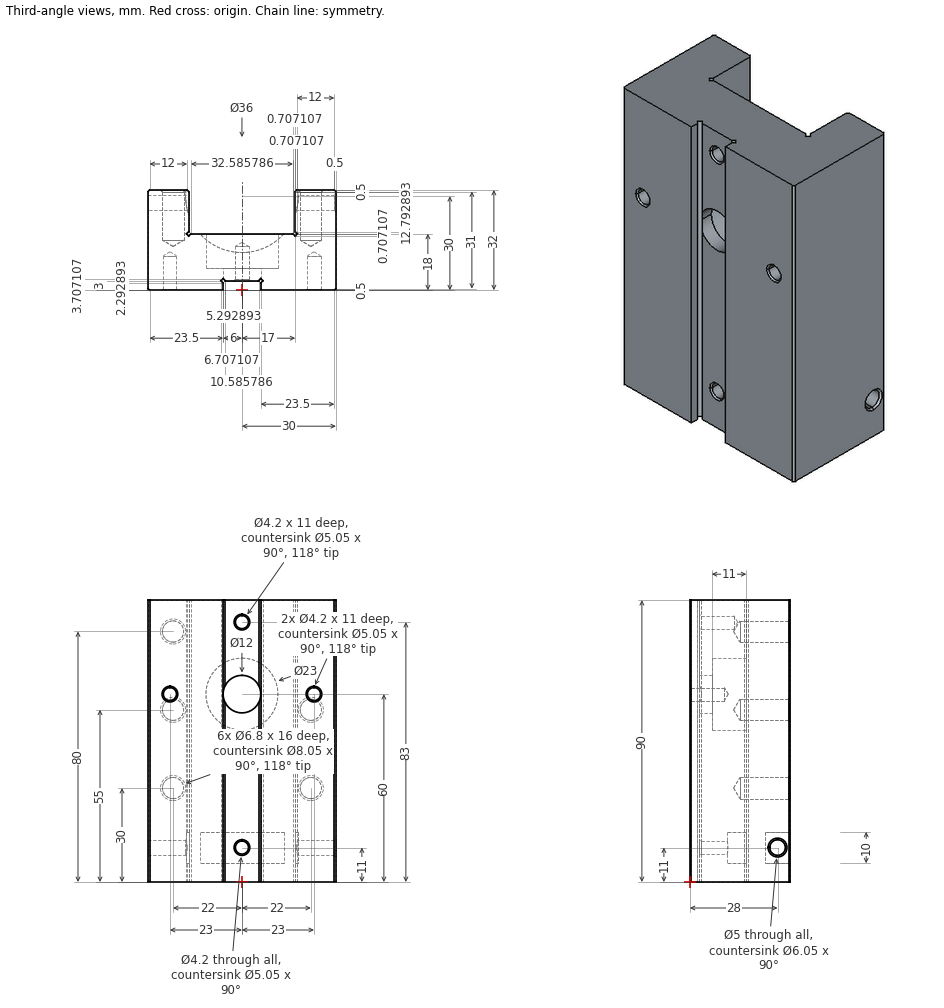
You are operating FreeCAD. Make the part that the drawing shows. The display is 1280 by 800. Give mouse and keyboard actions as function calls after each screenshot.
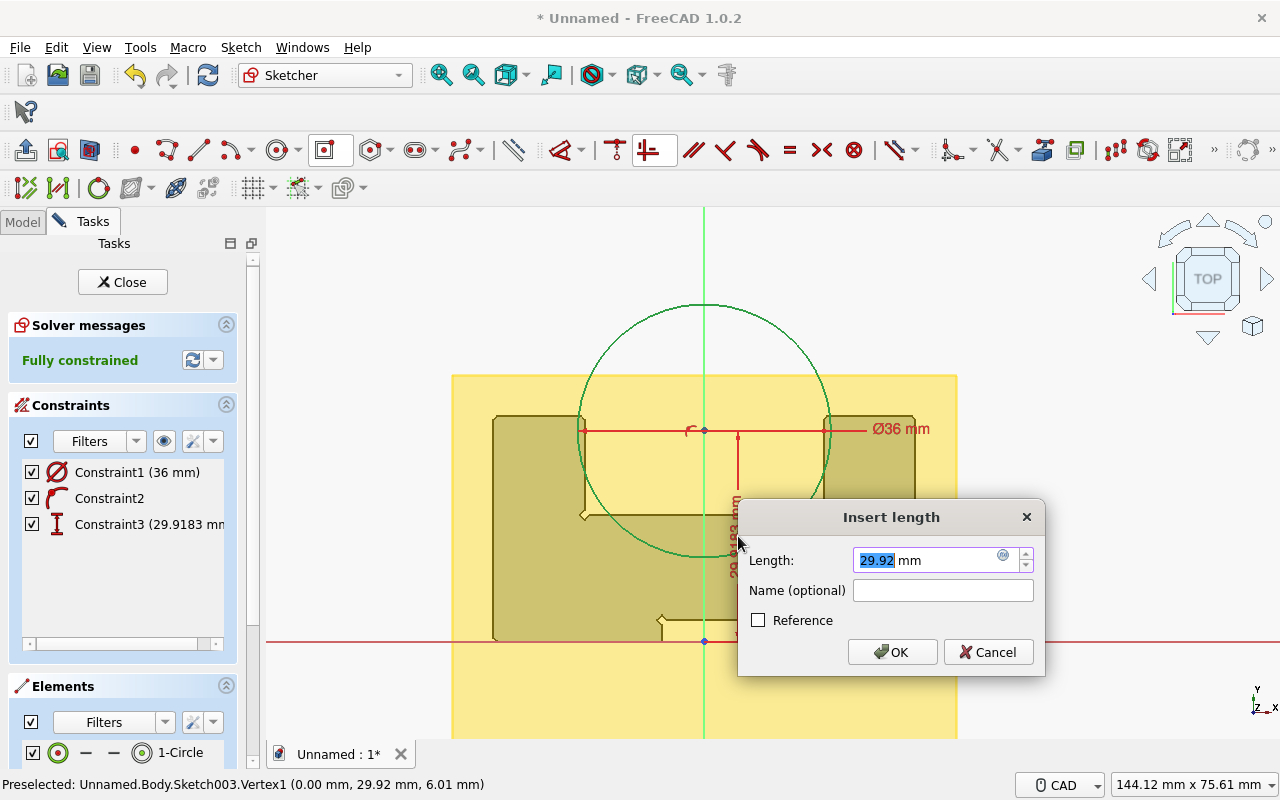
text(30)
key(Return)
key(Escape)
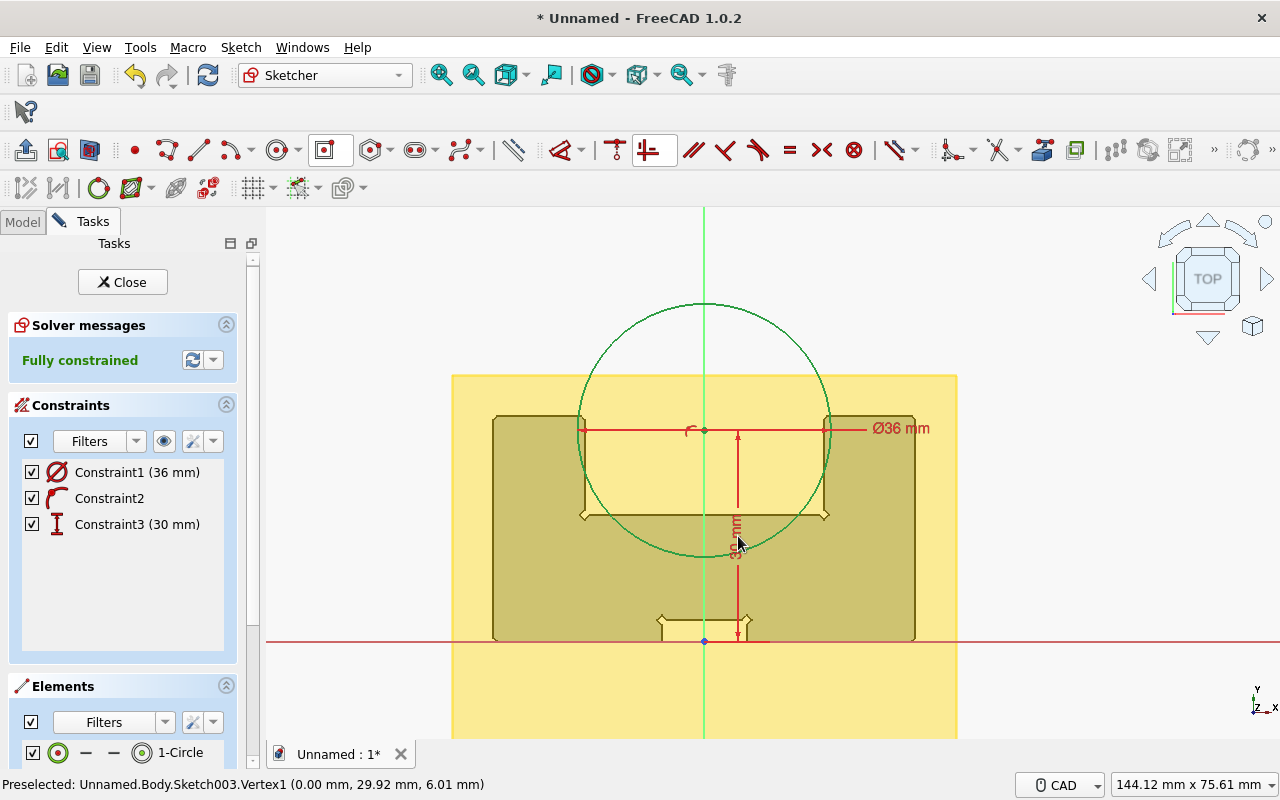
click(123, 282)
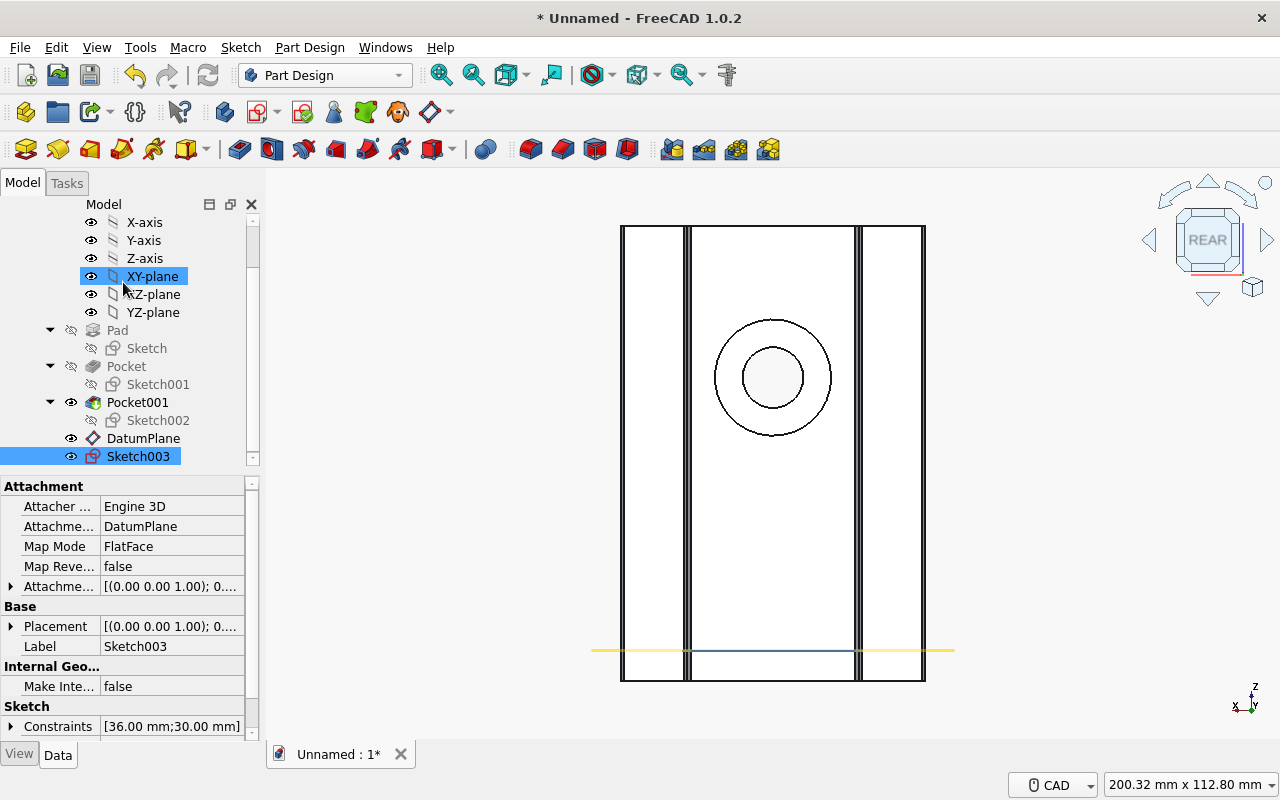
click(240, 150)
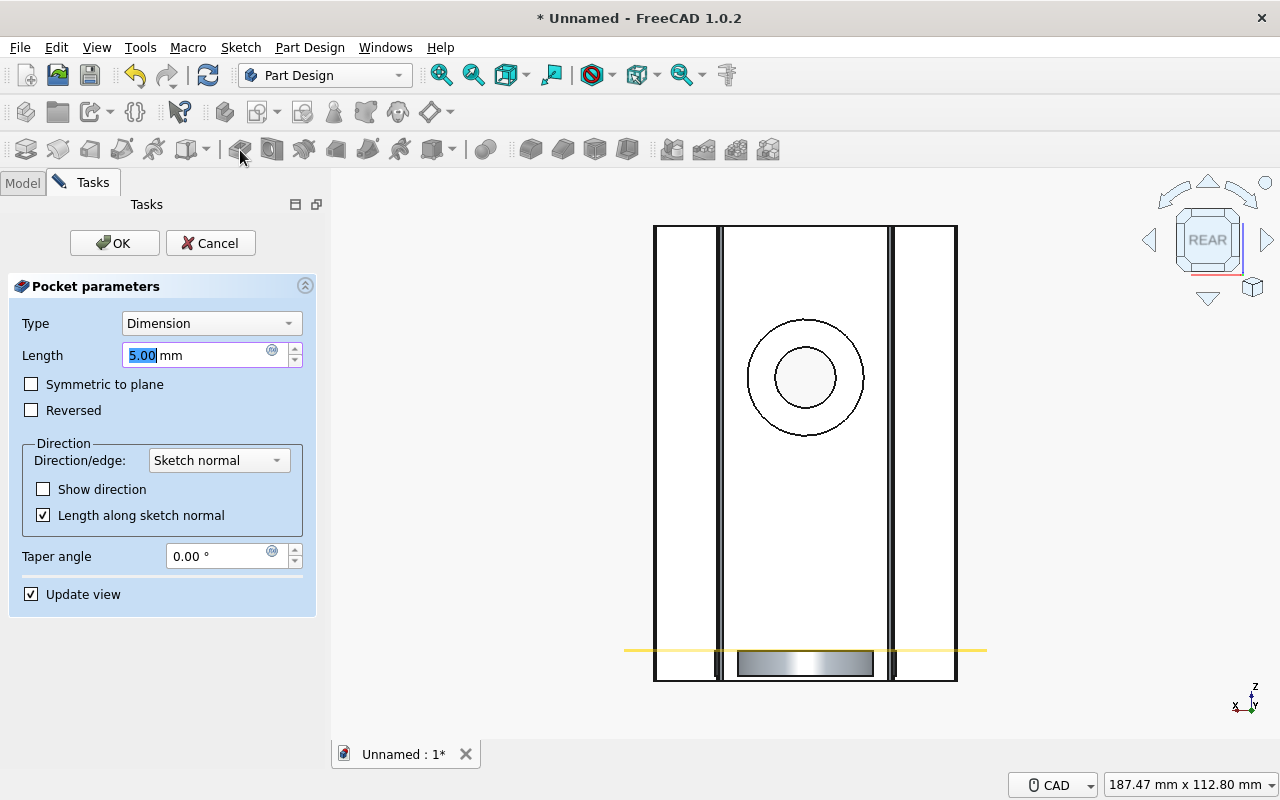
text(10)
key(Tab)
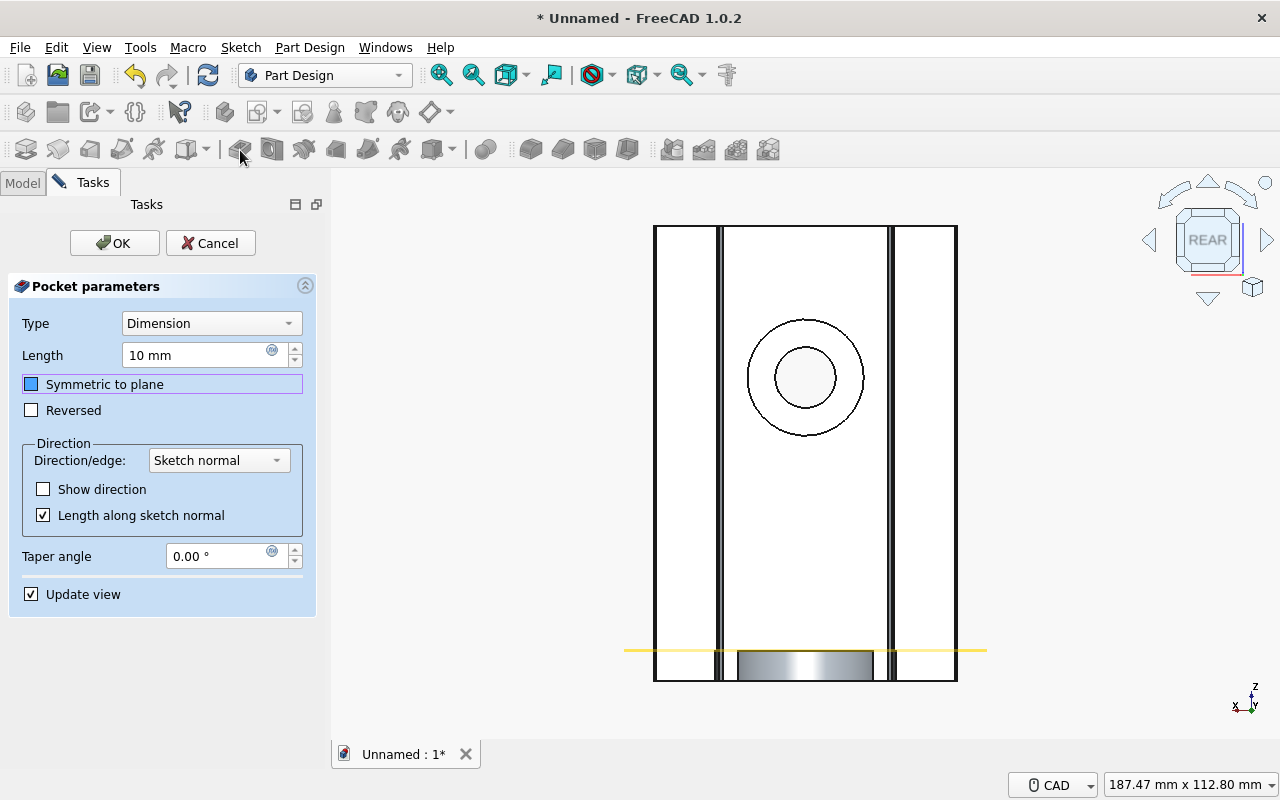
click(30, 410)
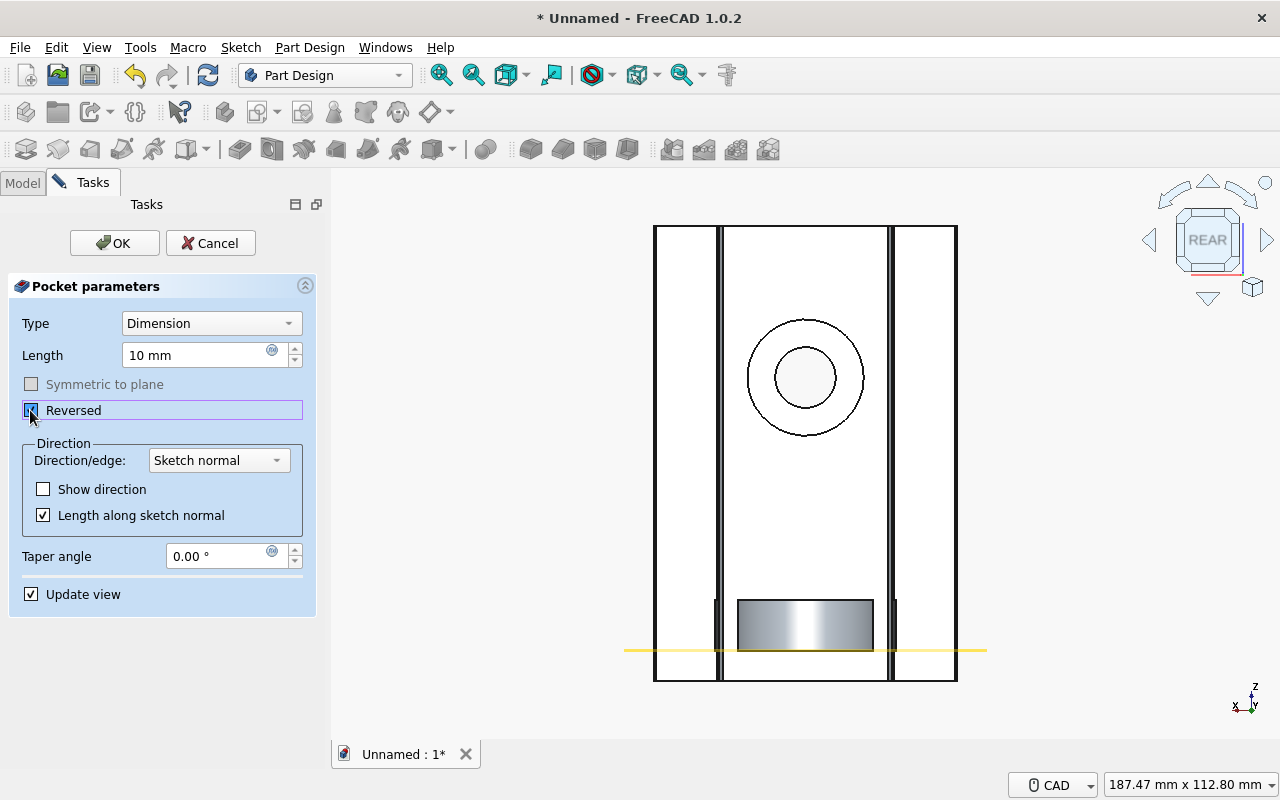
click(115, 243)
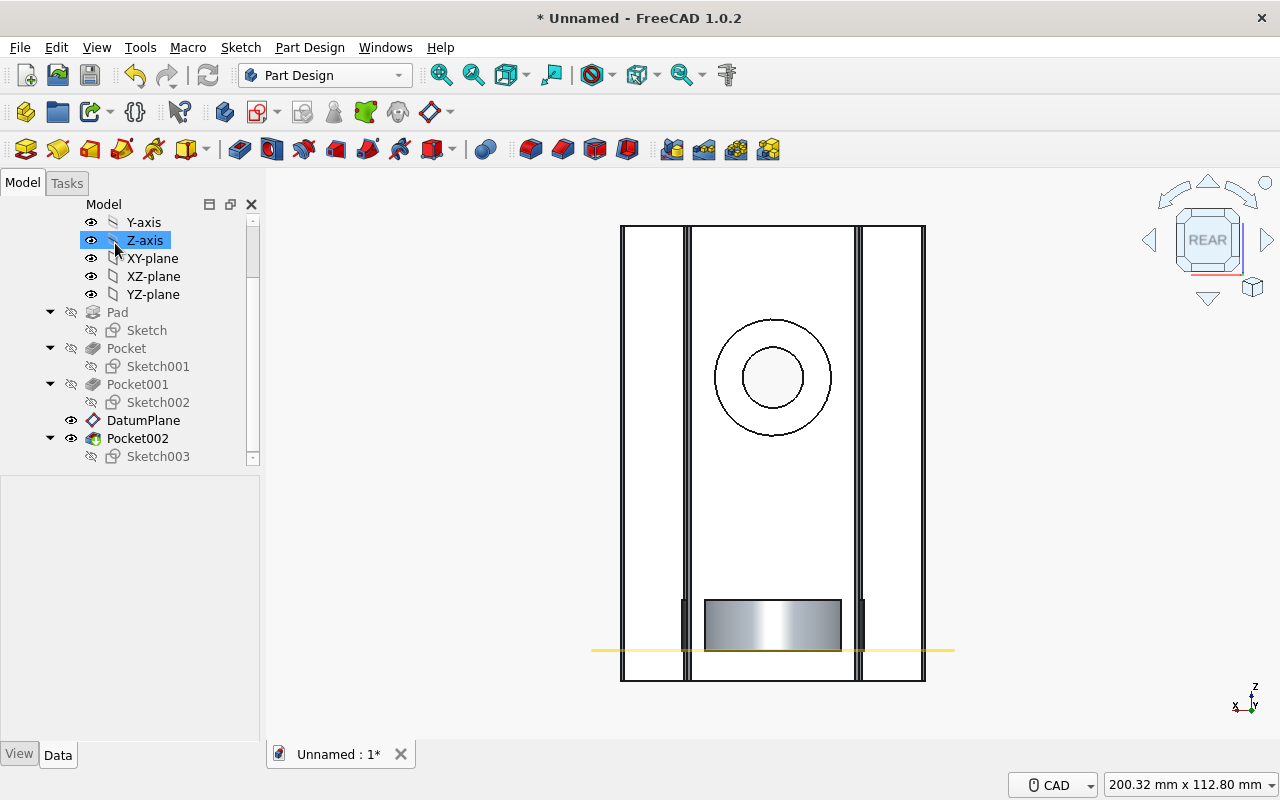
click(116, 420)
key(space)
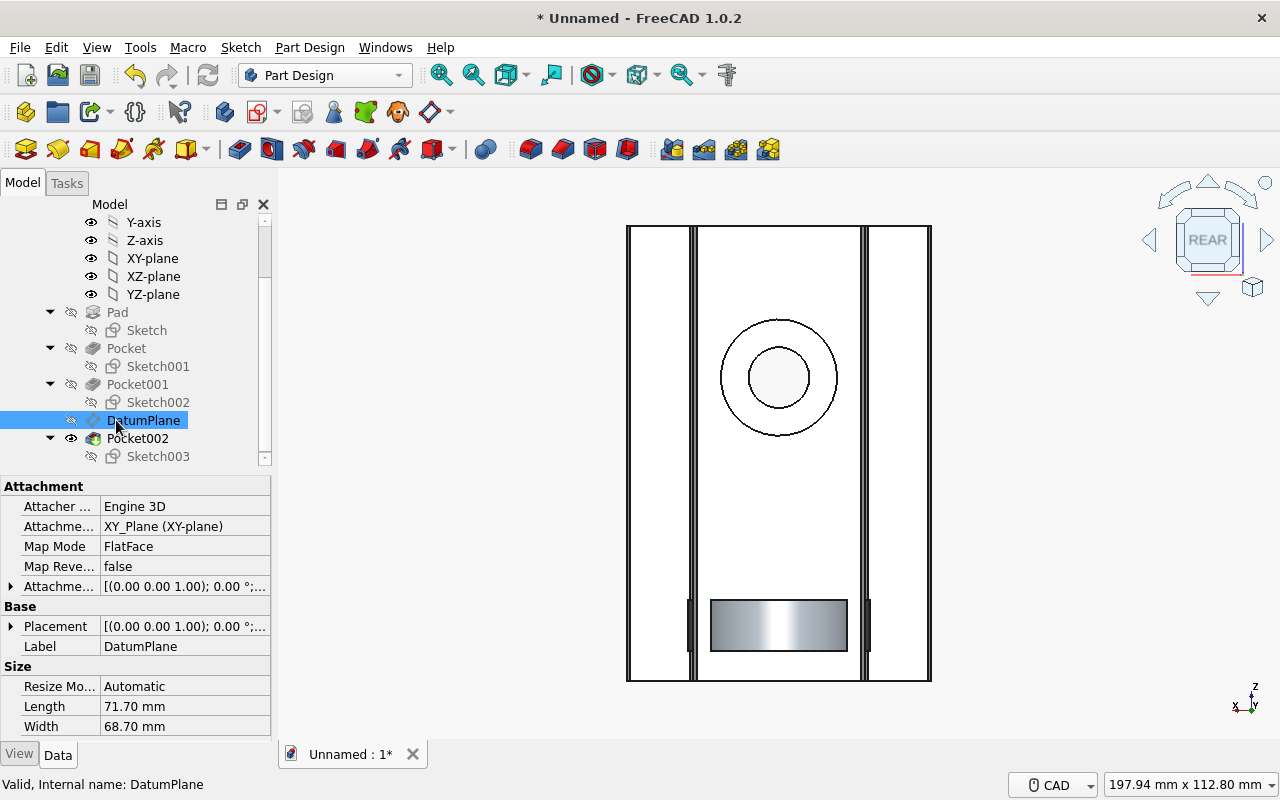
click(898, 257)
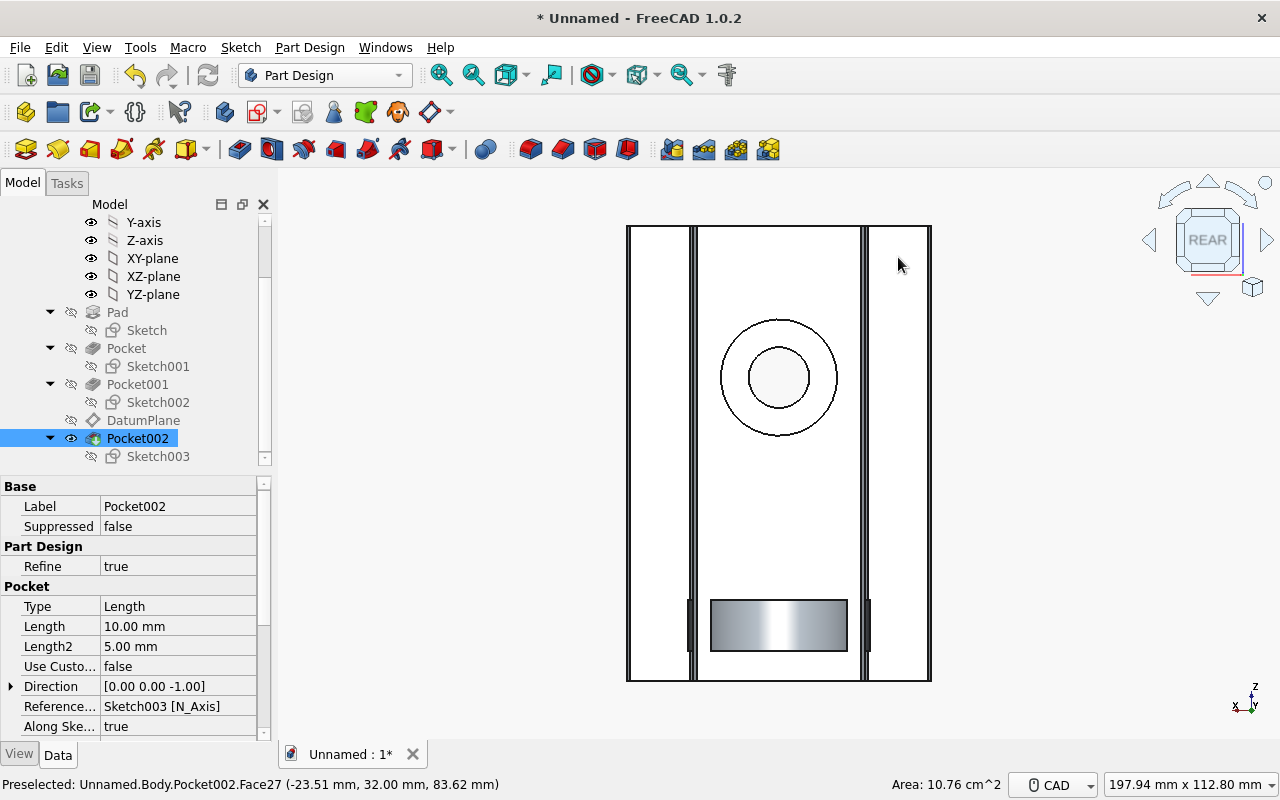
click(258, 112)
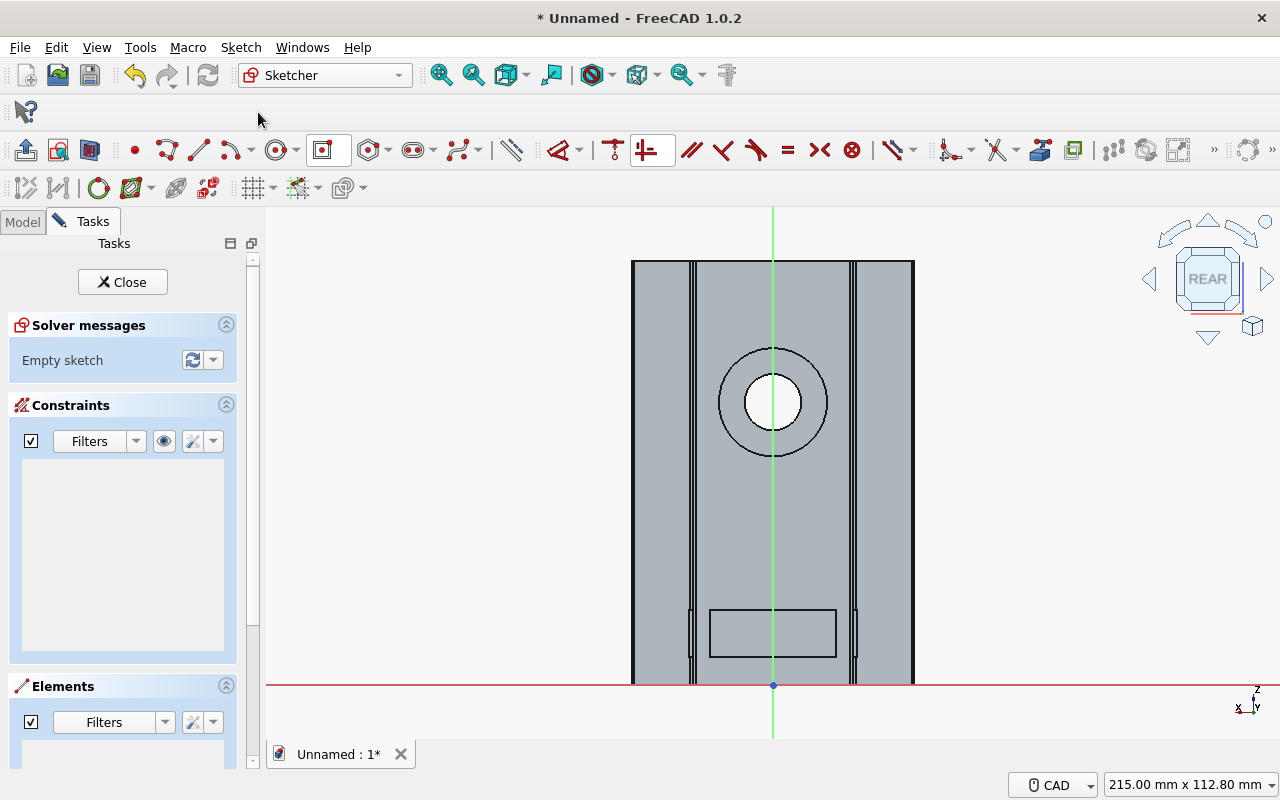
click(276, 150)